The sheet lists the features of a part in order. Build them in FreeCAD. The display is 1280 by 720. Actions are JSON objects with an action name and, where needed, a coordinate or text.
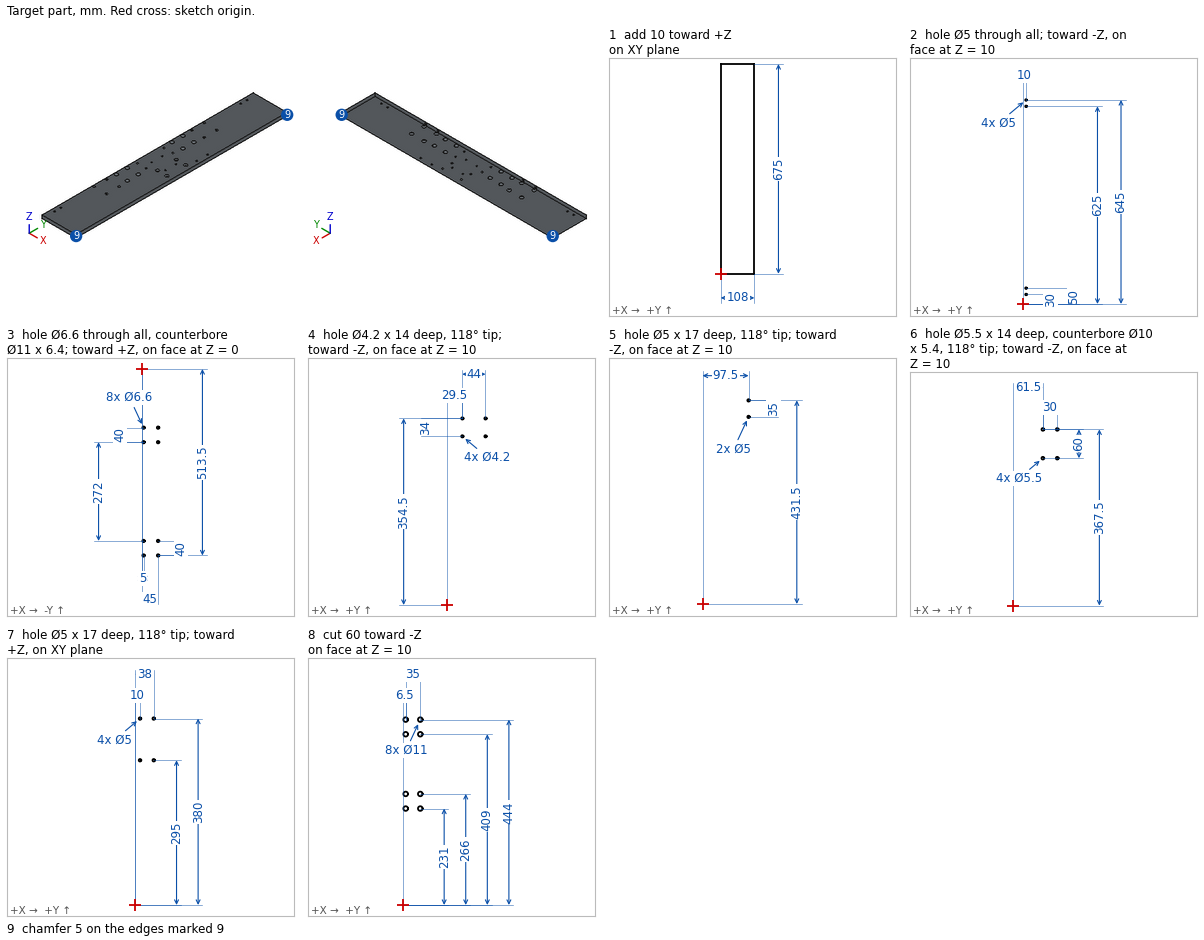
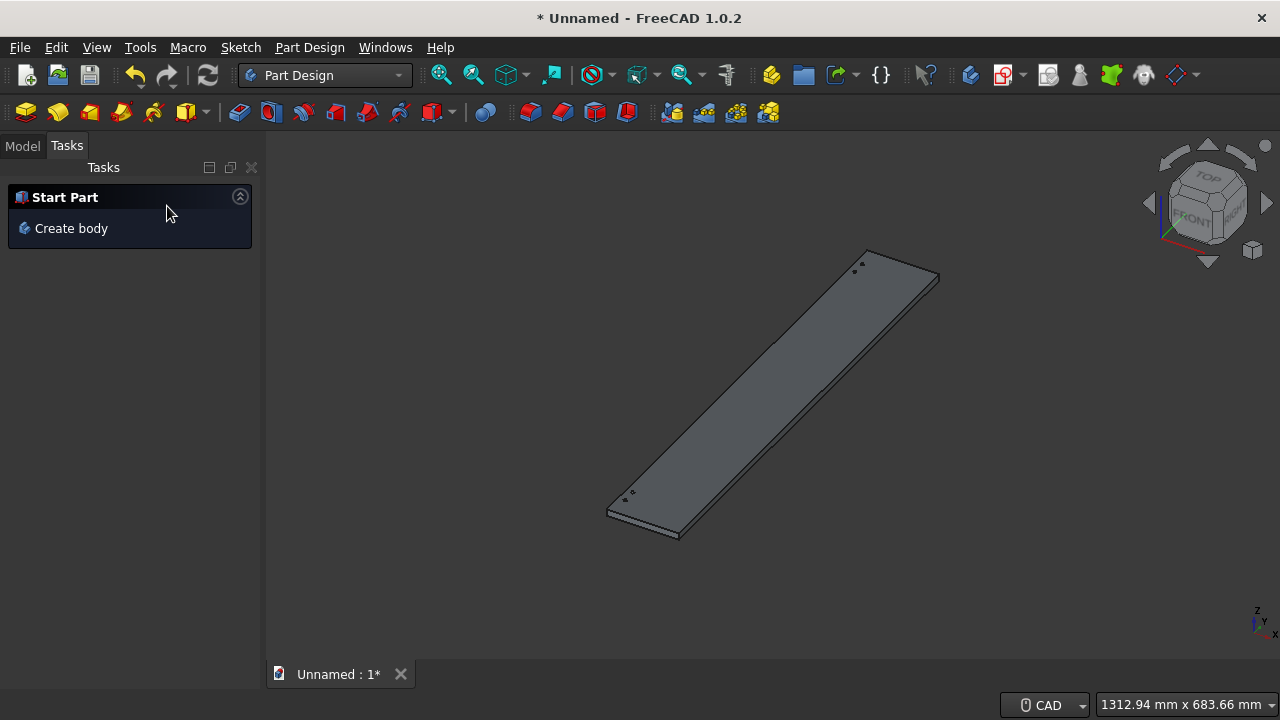
{"action": "key", "text": "5"}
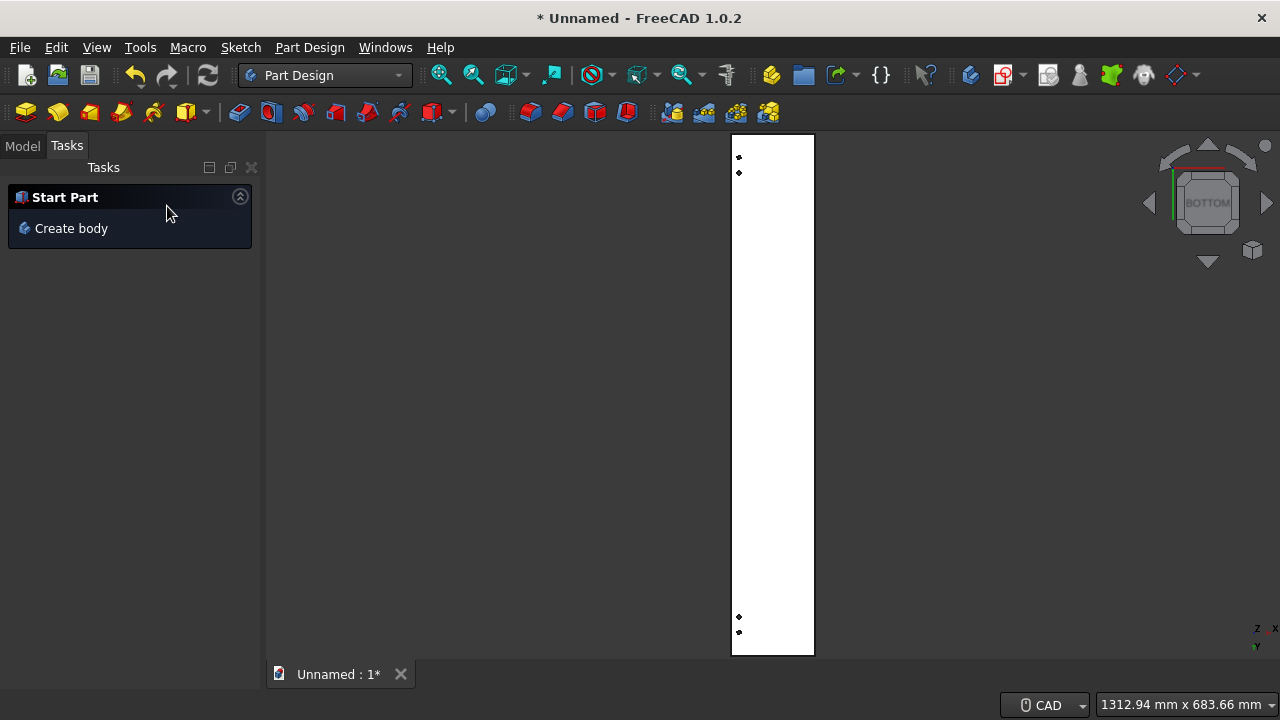
{"action": "left_click", "coordinate": [773, 543]}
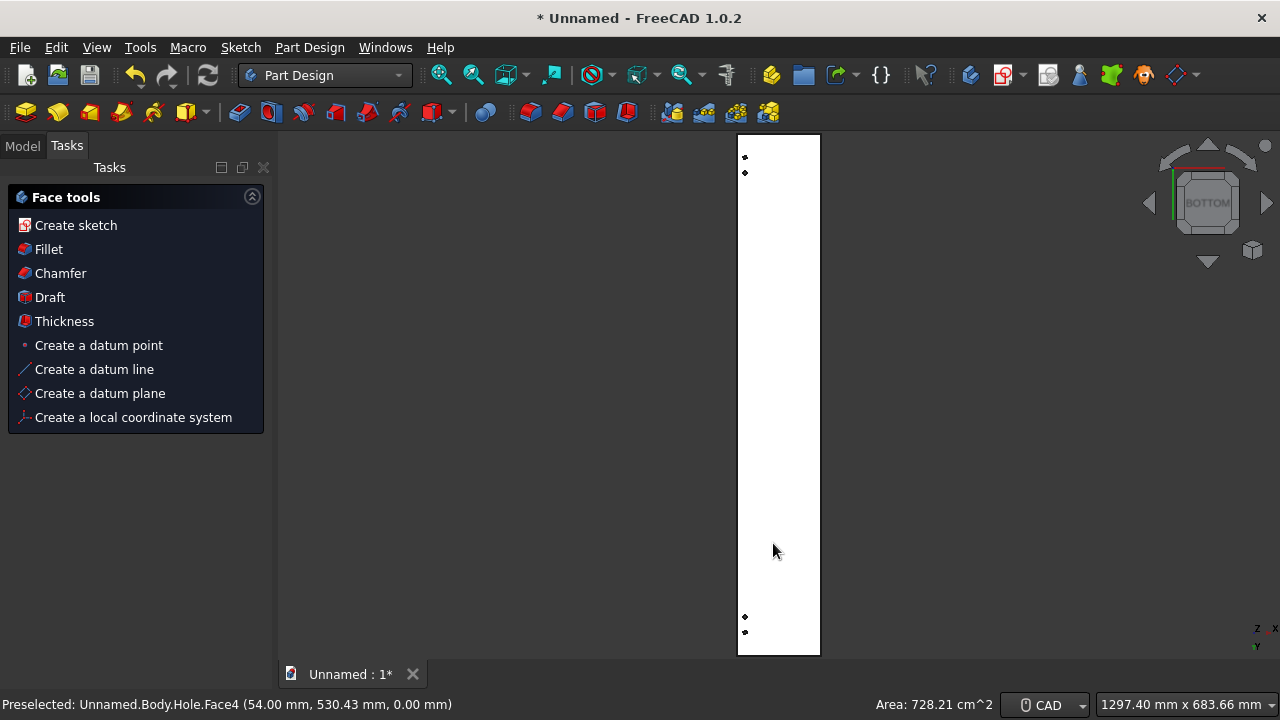
{"action": "left_click", "coordinate": [1004, 76]}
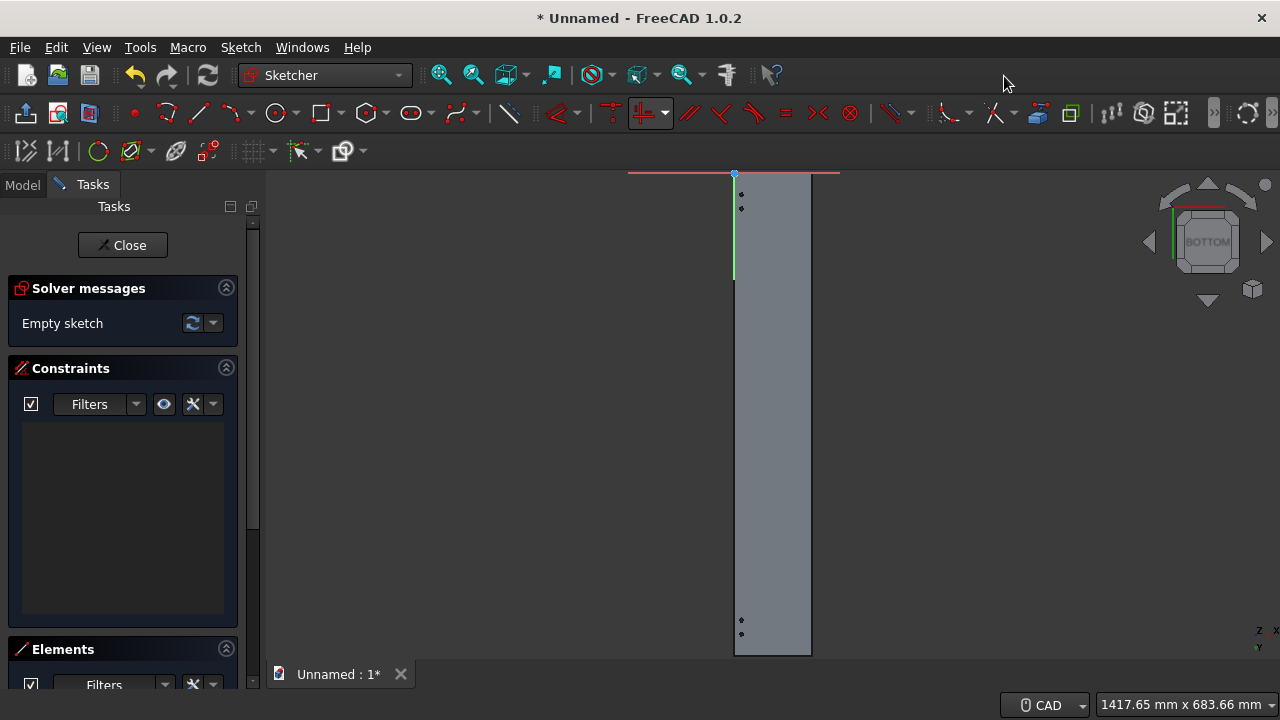
{"action": "scroll", "coordinate": [492, 631], "scroll_direction": "down", "scroll_amount": 1}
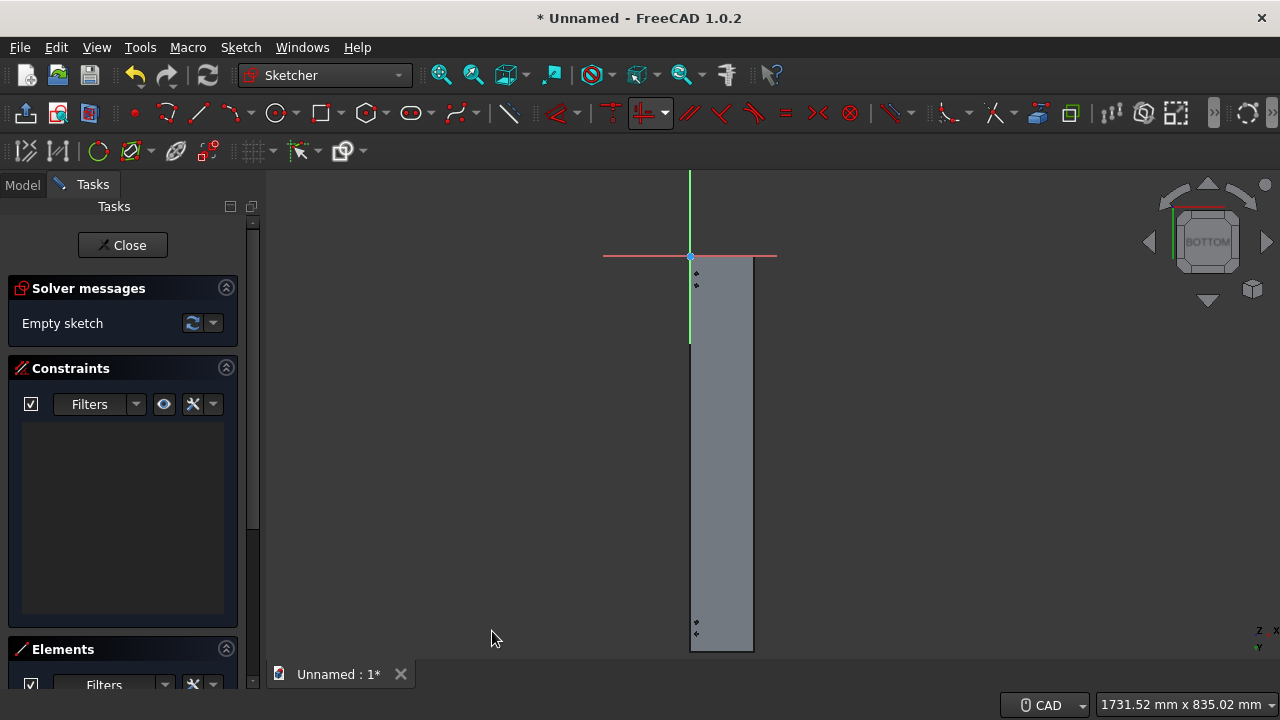
{"action": "left_click", "coordinate": [276, 114]}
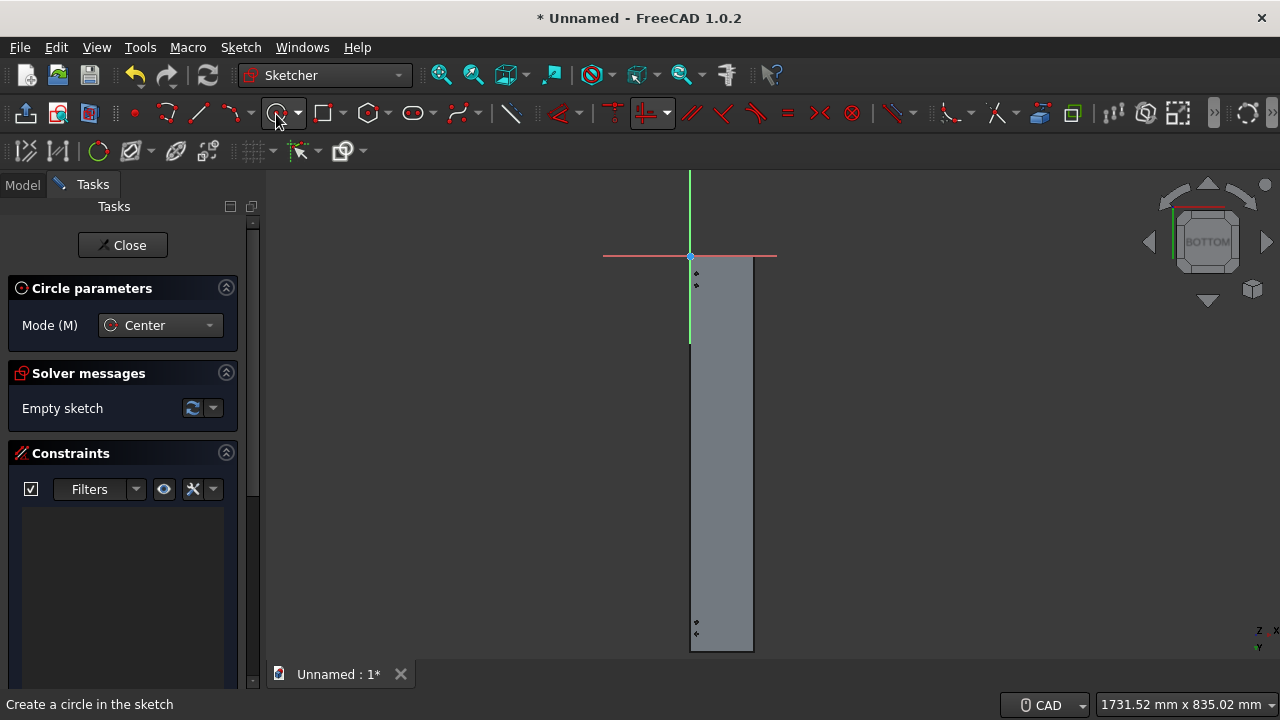
{"action": "scroll", "coordinate": [717, 557], "scroll_direction": "up", "scroll_amount": 13}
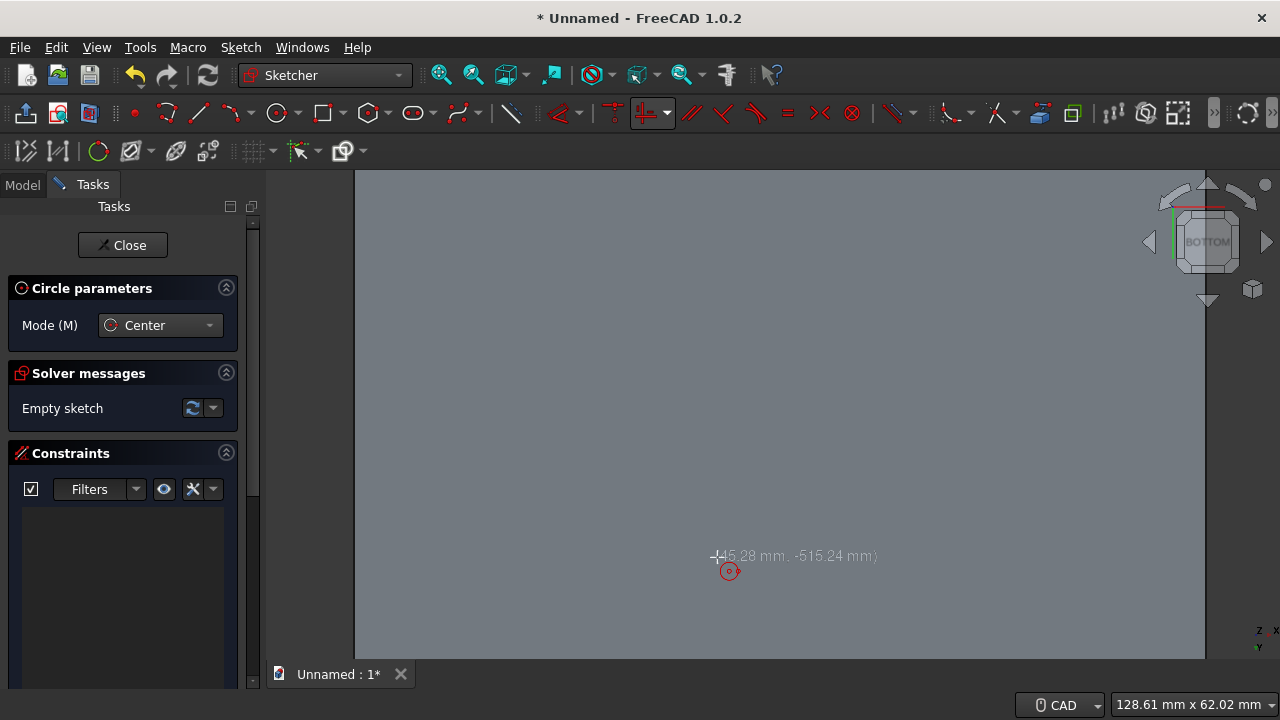
{"action": "scroll", "coordinate": [717, 565], "scroll_direction": "down", "scroll_amount": 13}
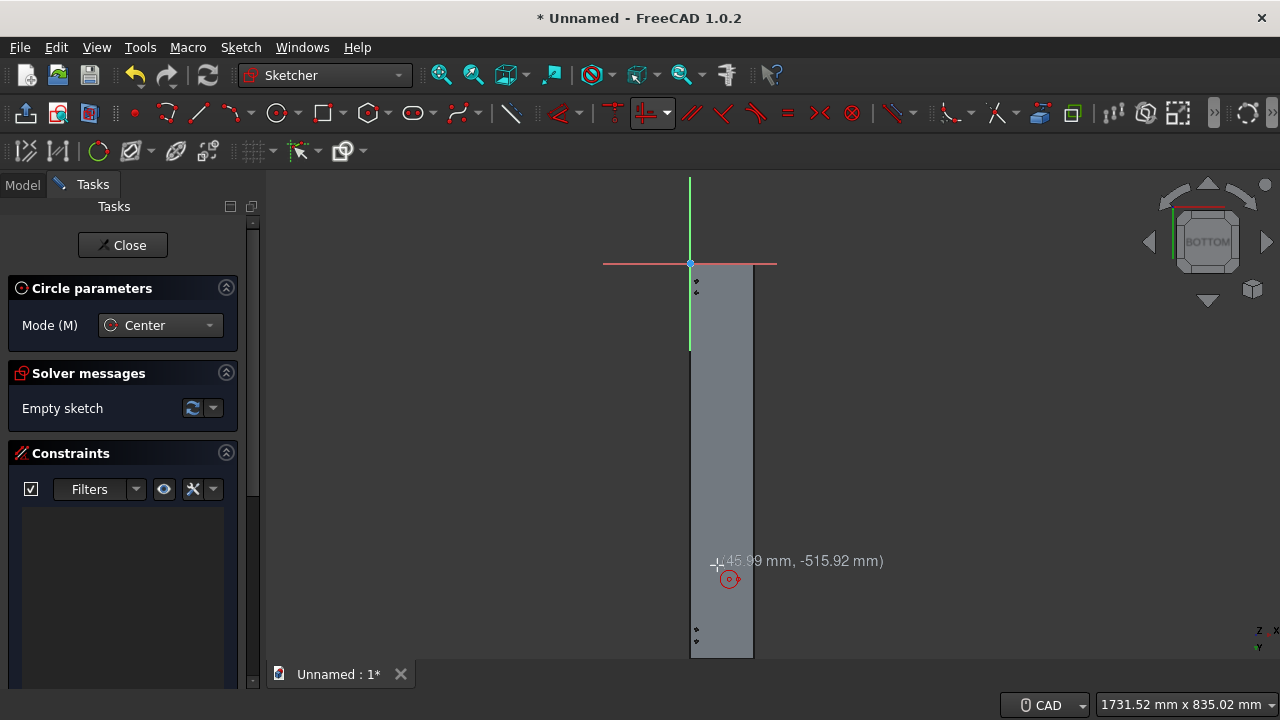
{"action": "left_click", "coordinate": [717, 564]}
{"action": "mouse_move", "coordinate": [718, 563]}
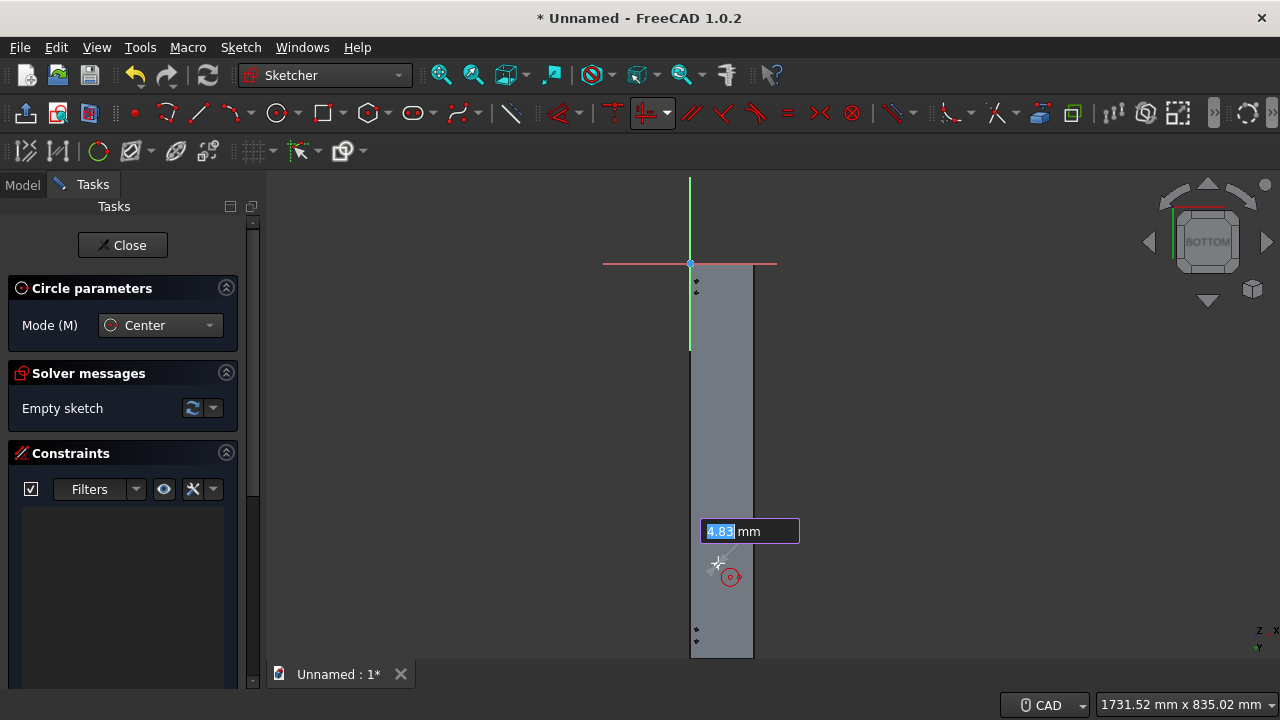
{"action": "type", "text": "6.6"}
{"action": "key", "text": "Return"}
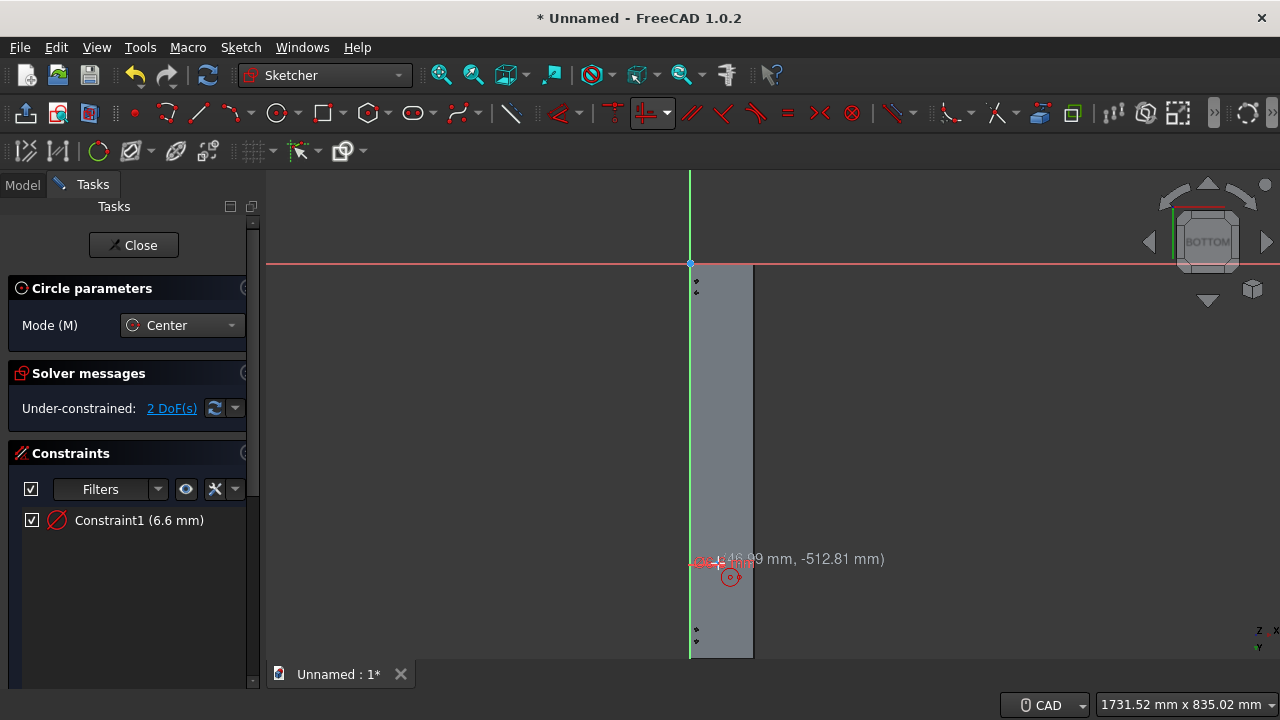
{"action": "scroll", "coordinate": [693, 564], "scroll_direction": "up", "scroll_amount": 13}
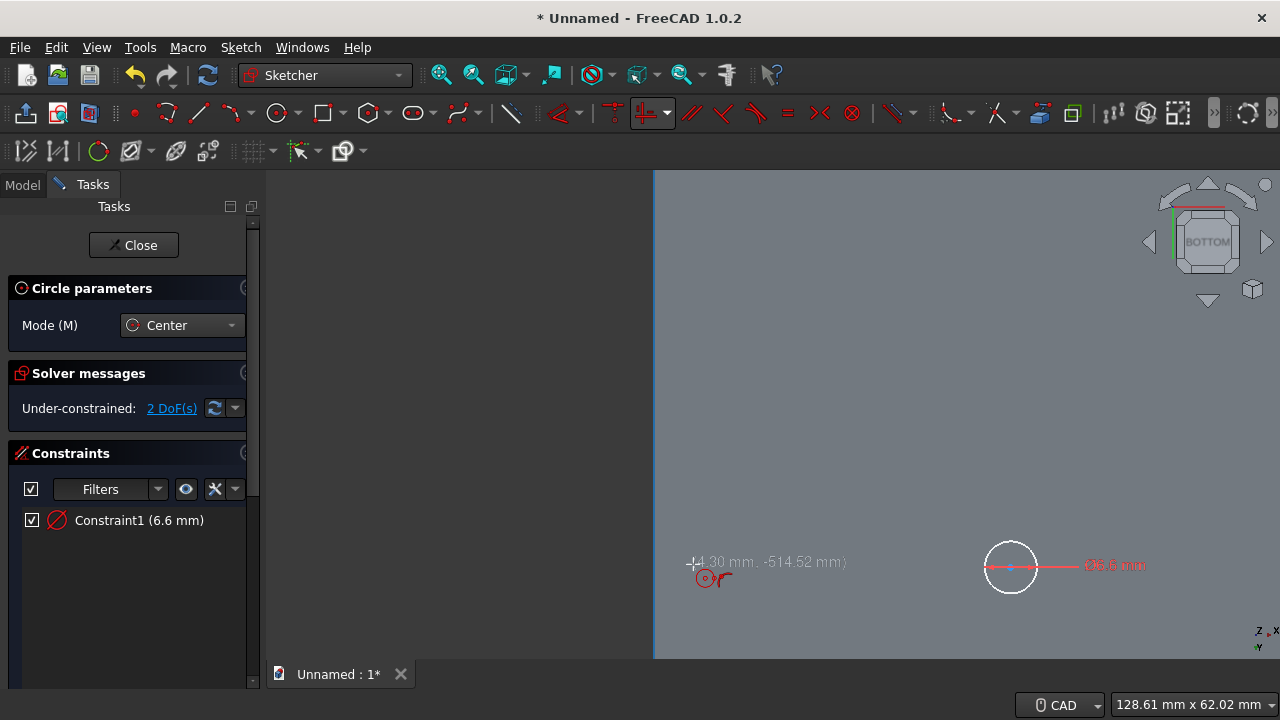
{"action": "left_click", "coordinate": [693, 559]}